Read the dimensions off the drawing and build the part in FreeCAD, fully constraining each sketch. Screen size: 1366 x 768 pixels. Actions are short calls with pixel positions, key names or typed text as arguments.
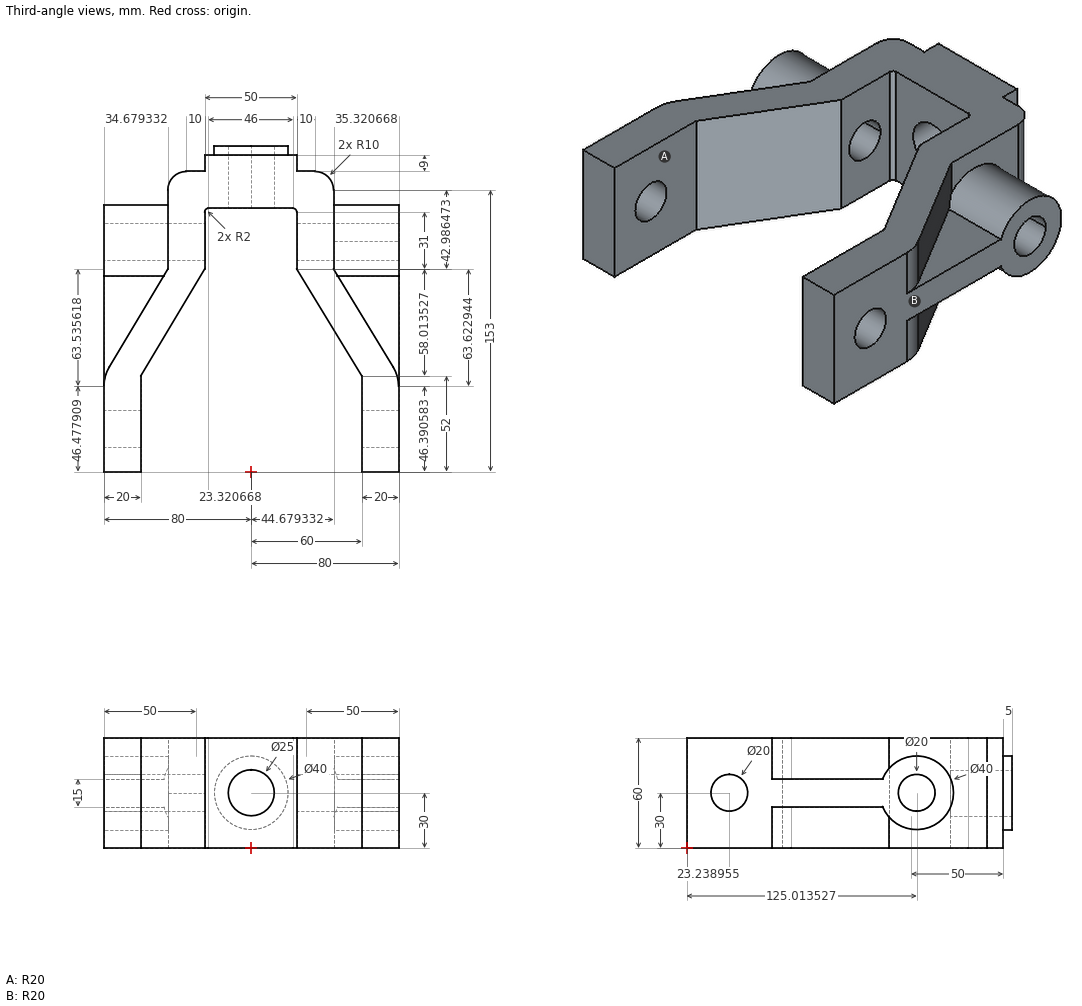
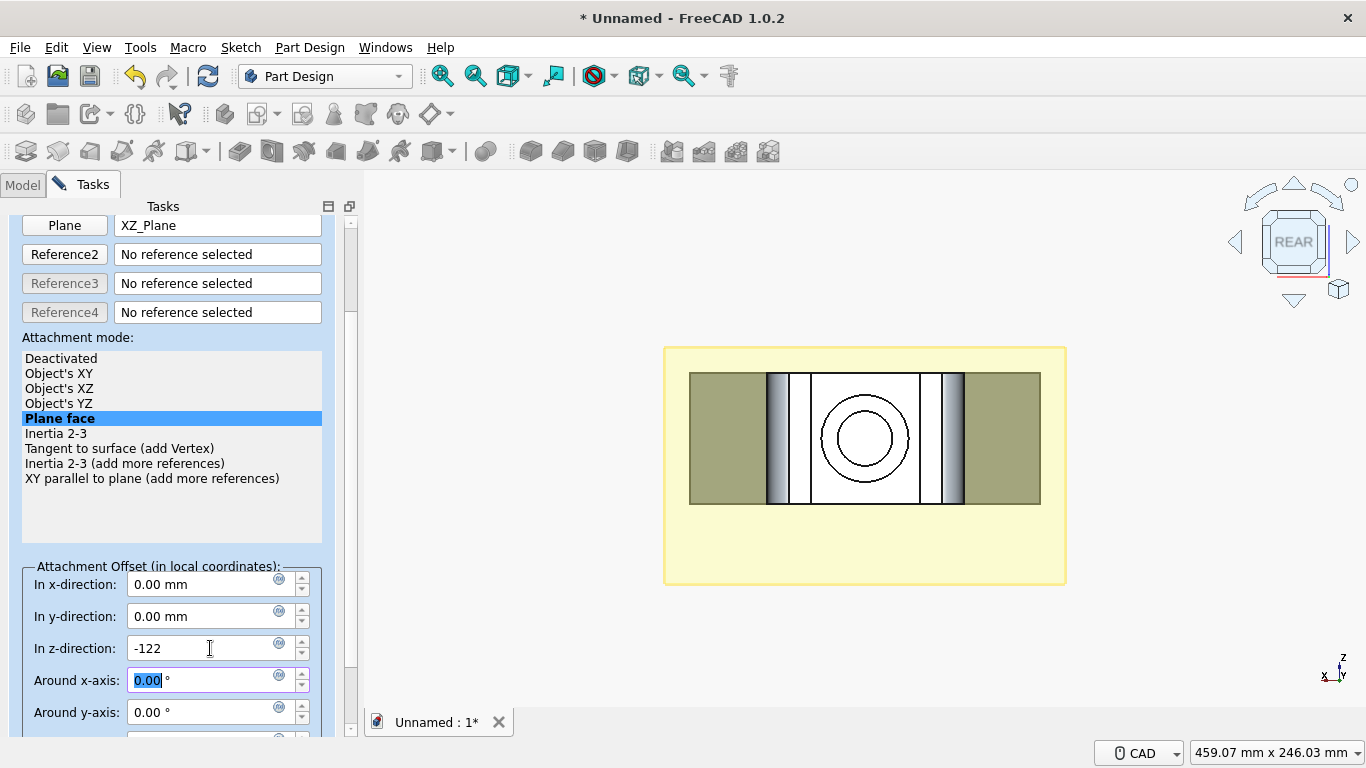
scroll(351, 476, up, 3)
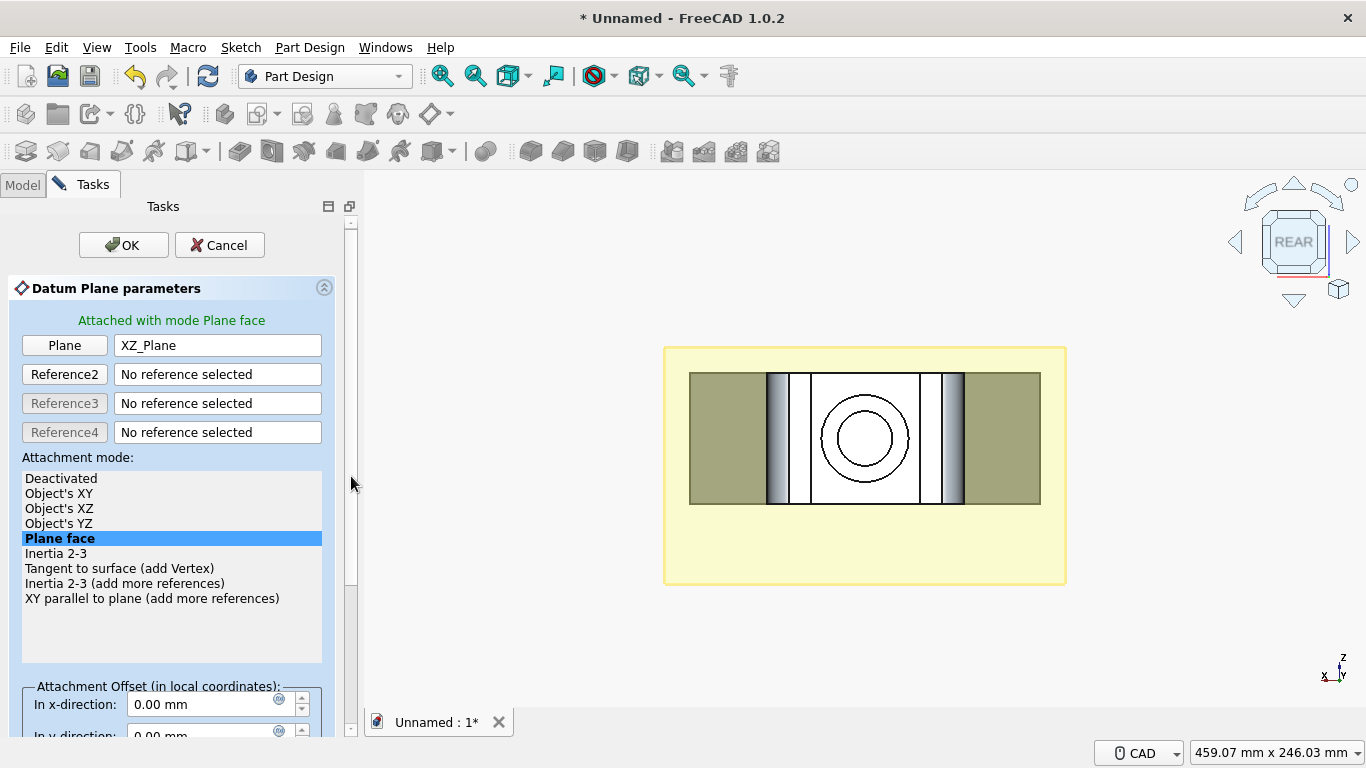
click(124, 245)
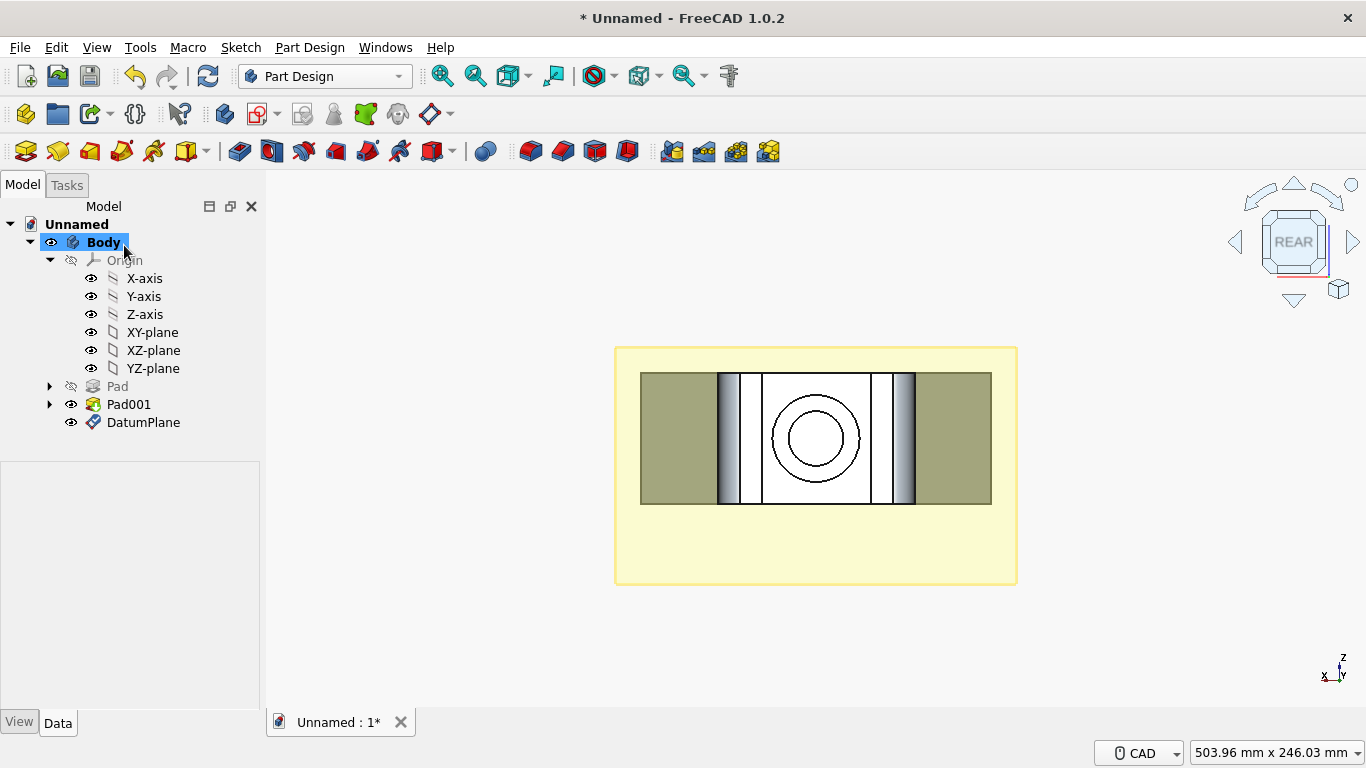
click(116, 422)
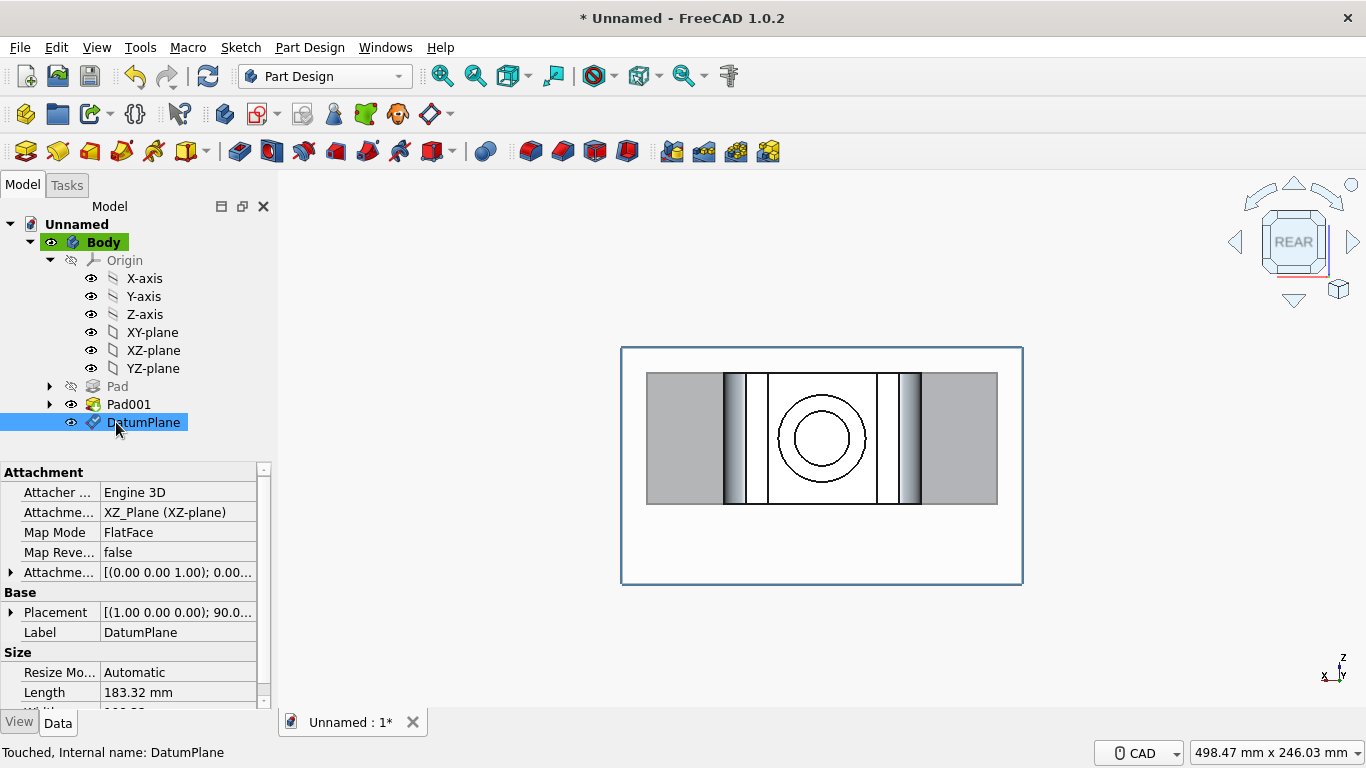
click(258, 114)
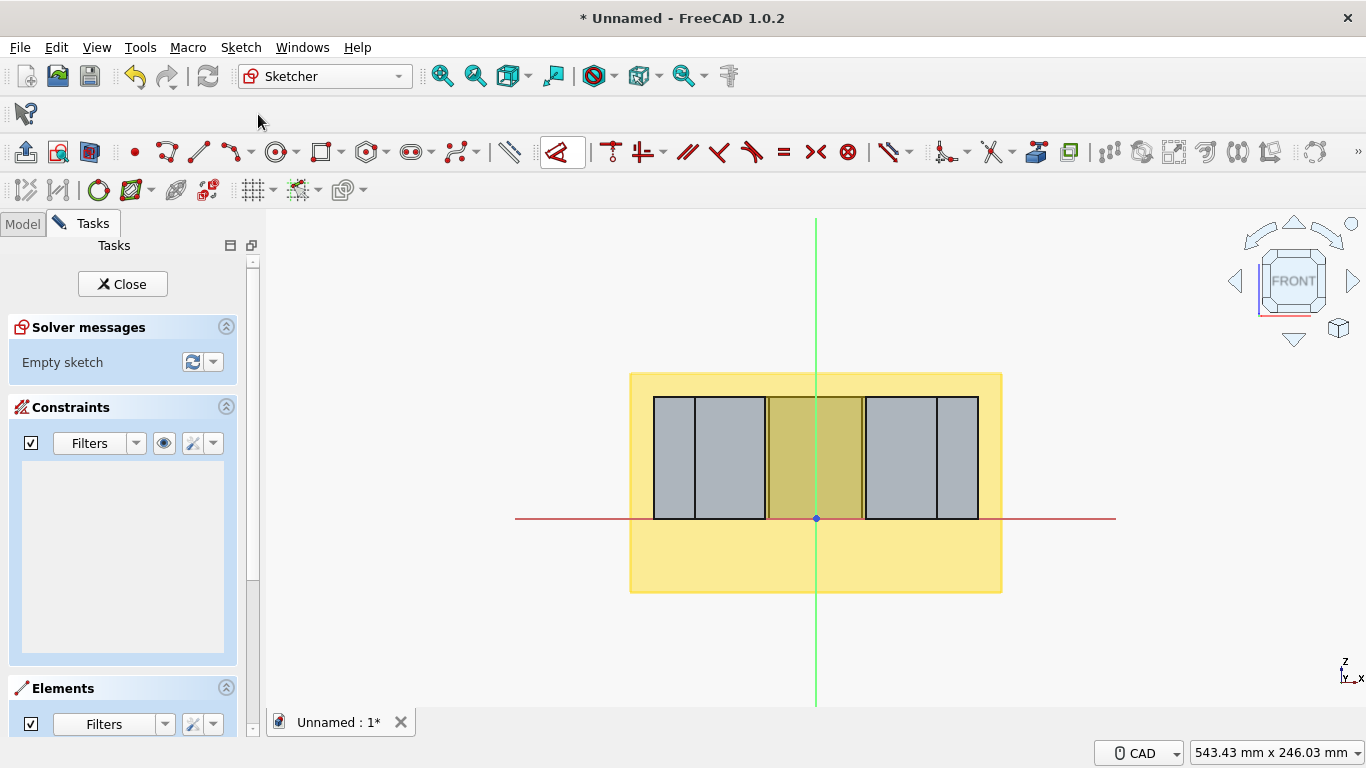
key(q)
key(s)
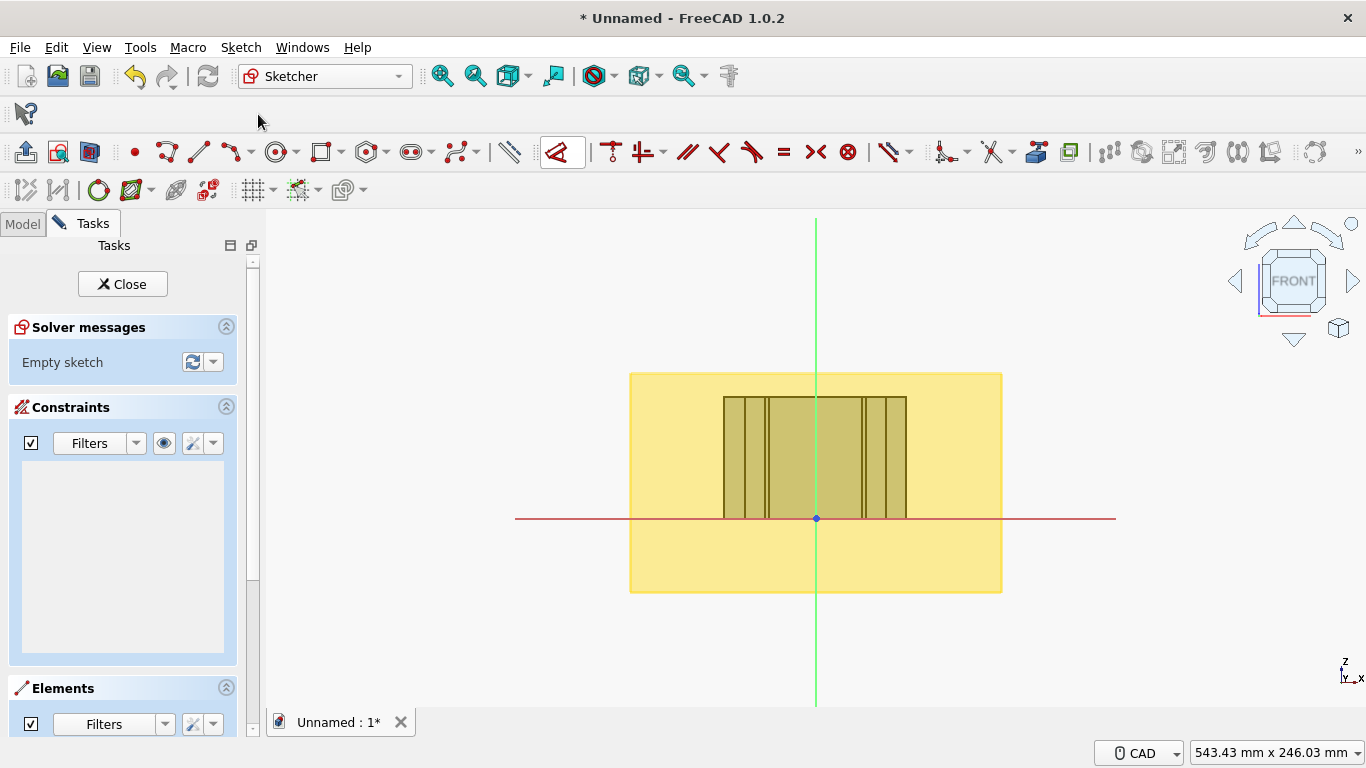
scroll(846, 483, up, 6)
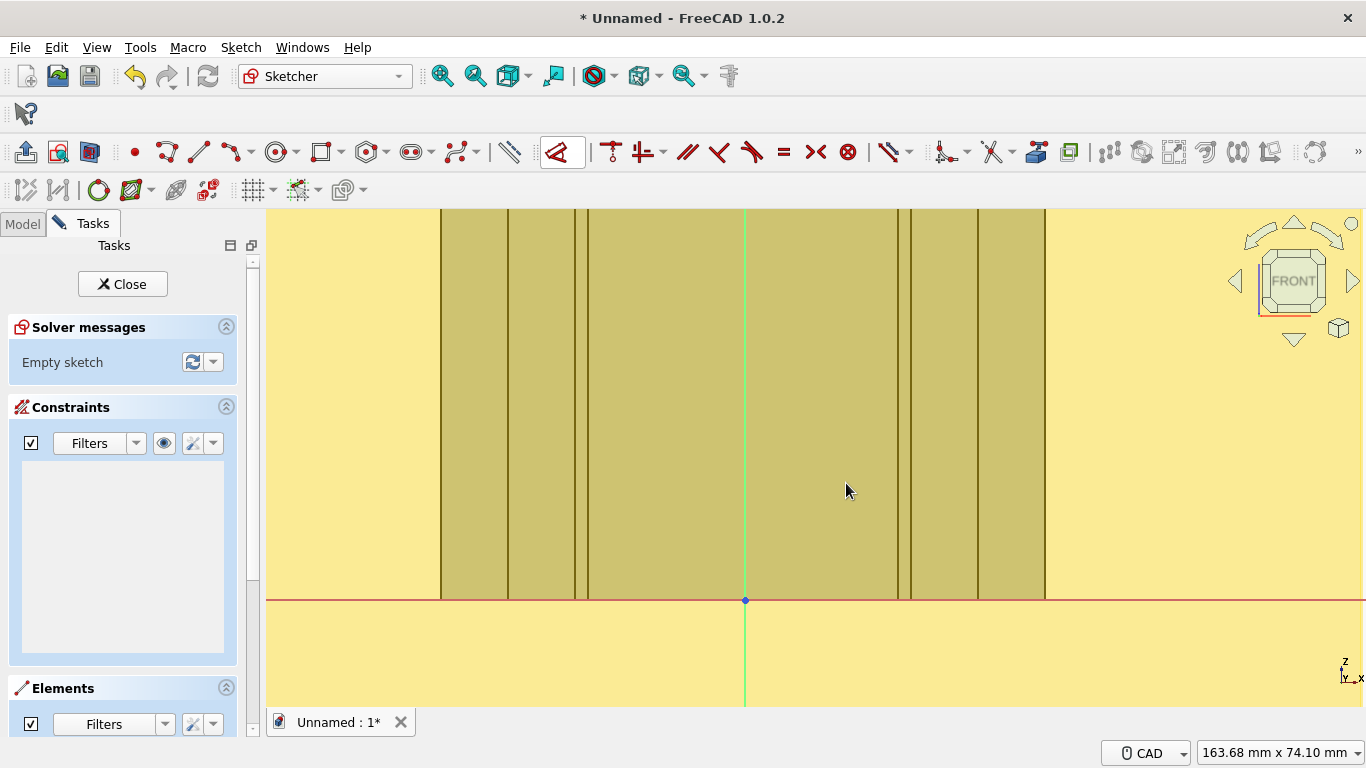
key(g)
key(c)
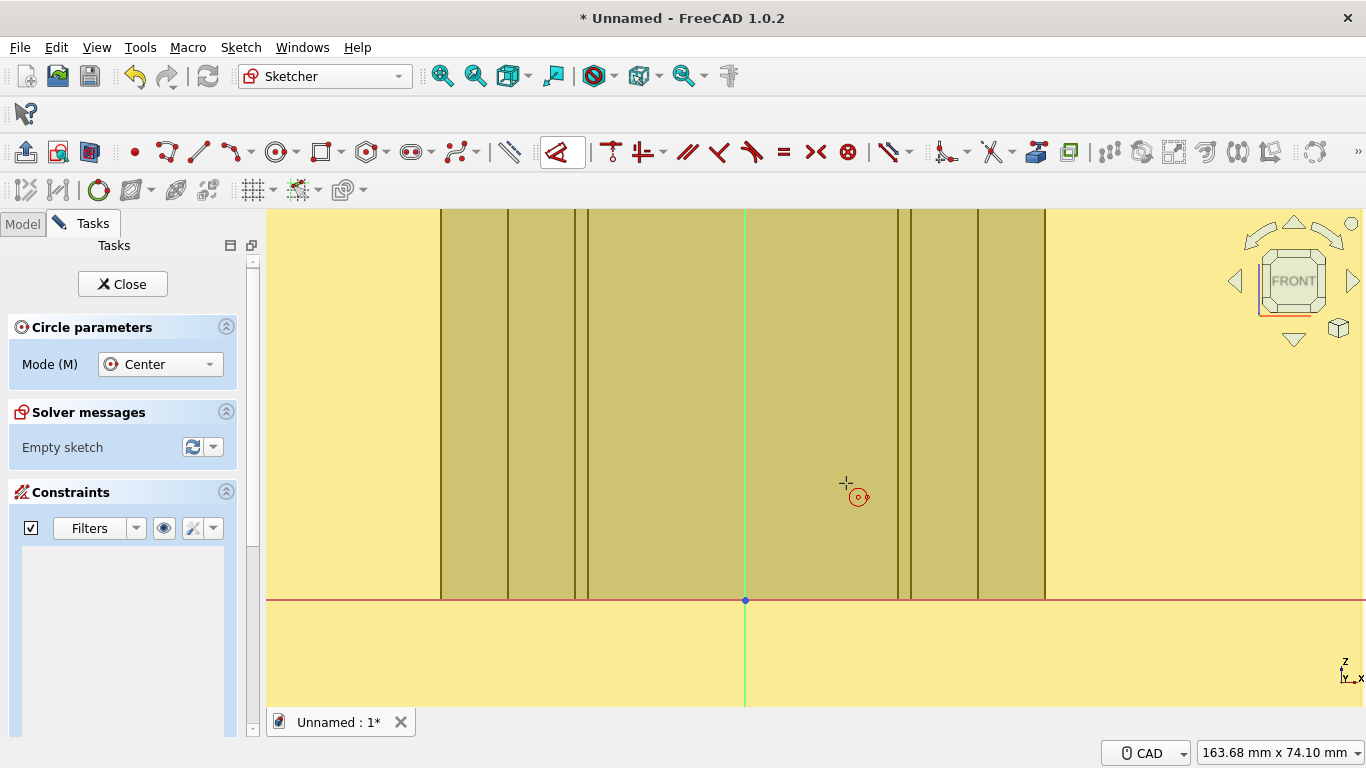
click(745, 399)
click(805, 339)
key(Escape)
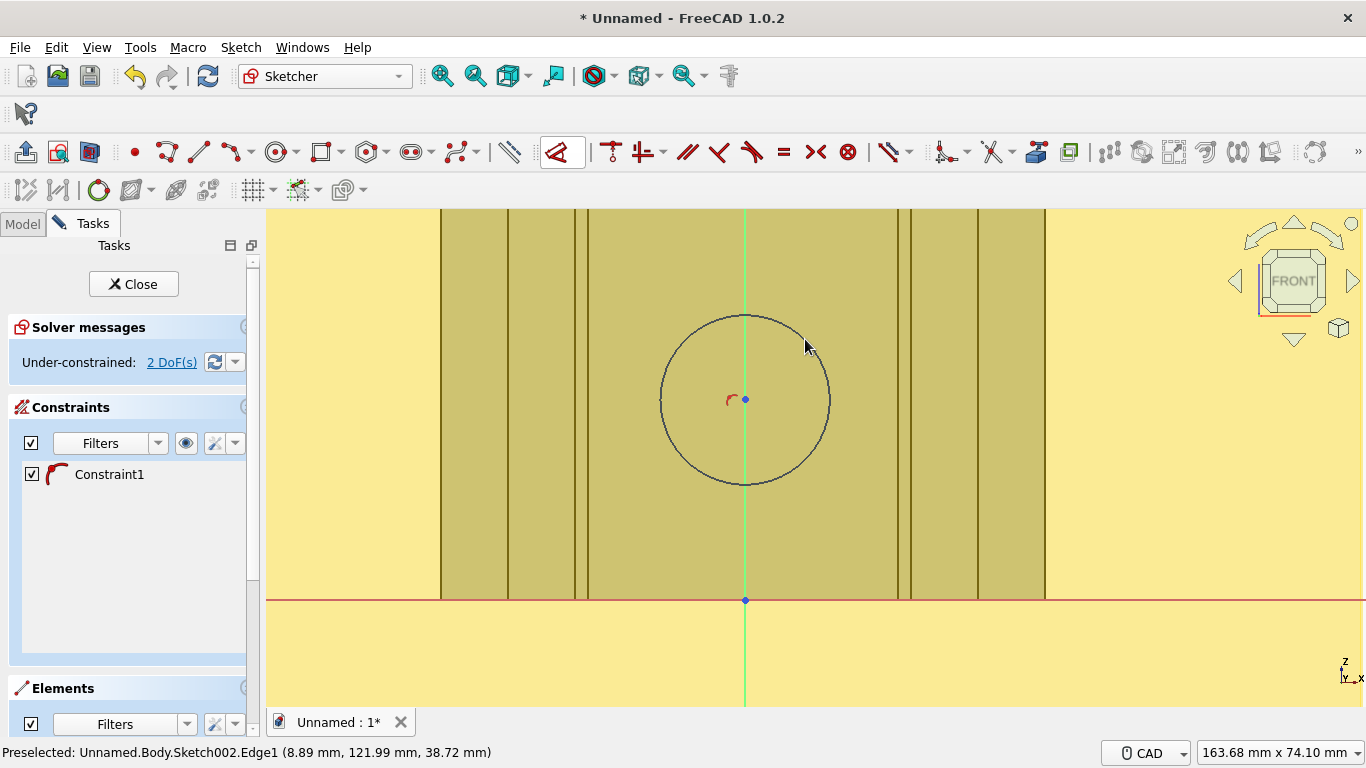
click(805, 340)